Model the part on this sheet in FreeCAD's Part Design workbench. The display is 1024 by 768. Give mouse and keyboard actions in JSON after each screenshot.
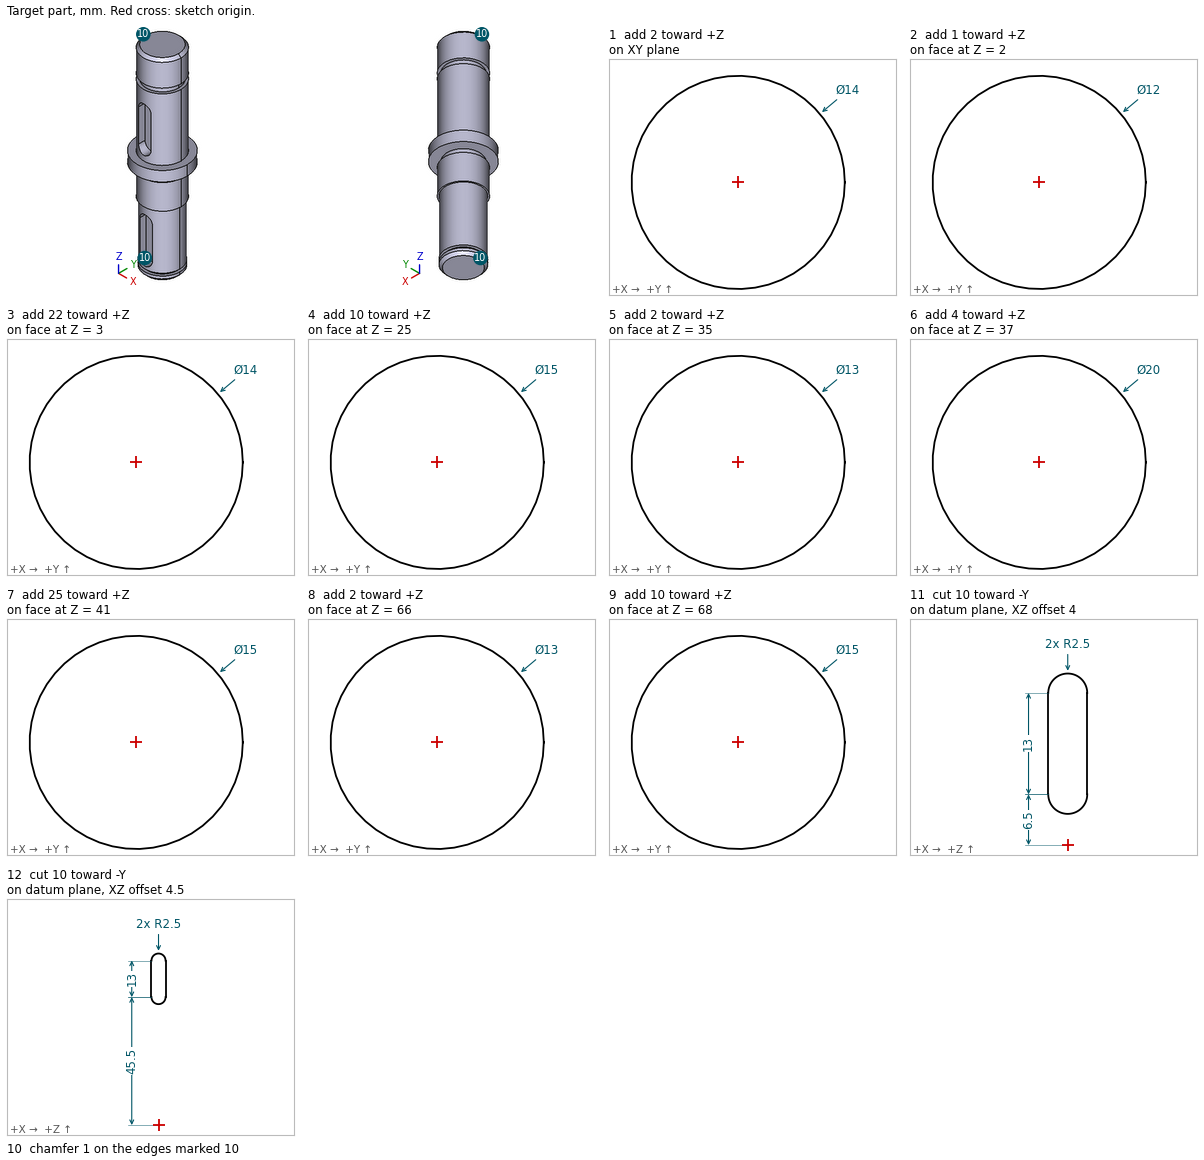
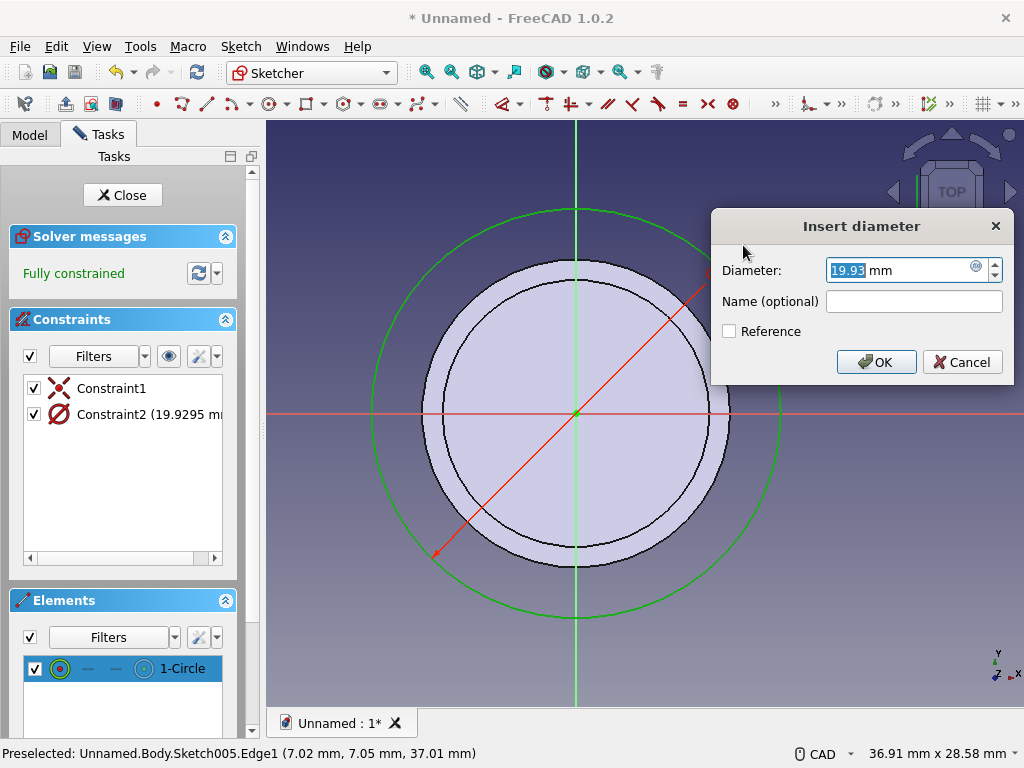
{"action": "type", "text": "20"}
{"action": "key", "text": "Return"}
{"action": "key", "text": "Escape"}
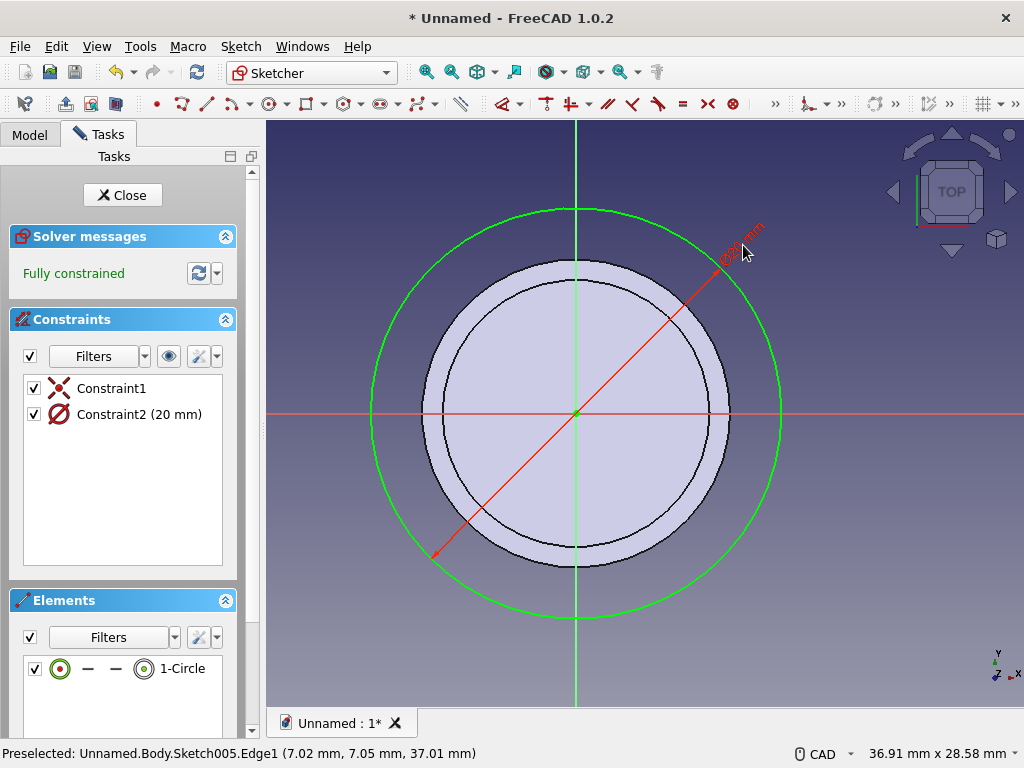
{"action": "left_click", "coordinate": [123, 195]}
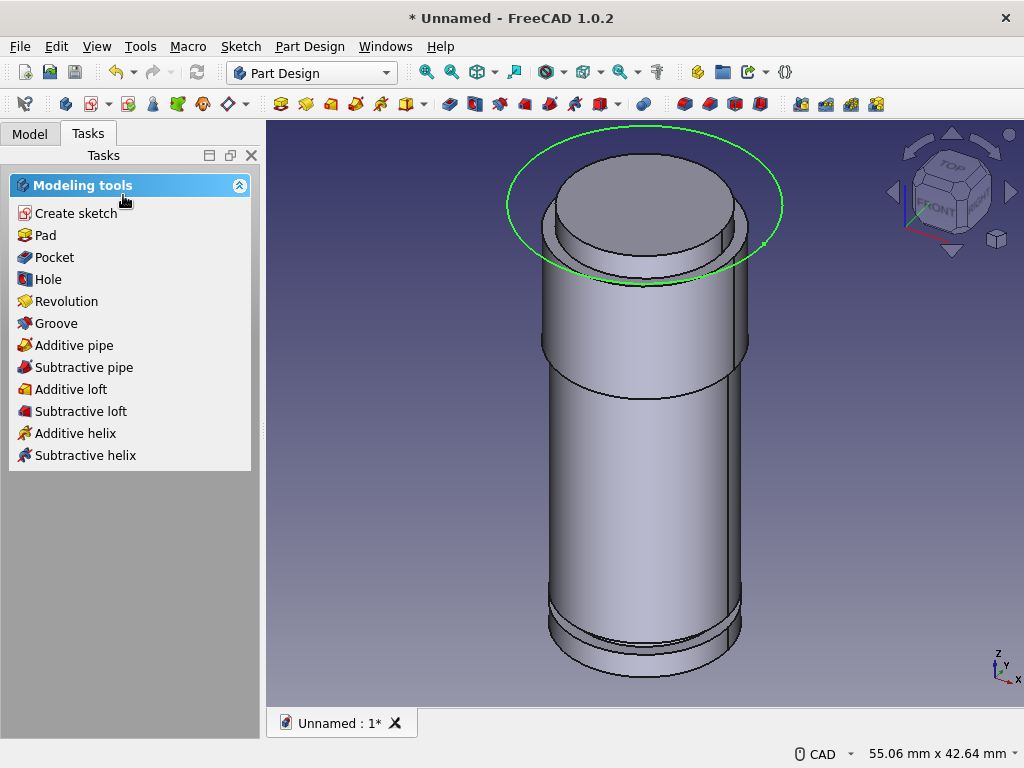
{"action": "left_click", "coordinate": [281, 104]}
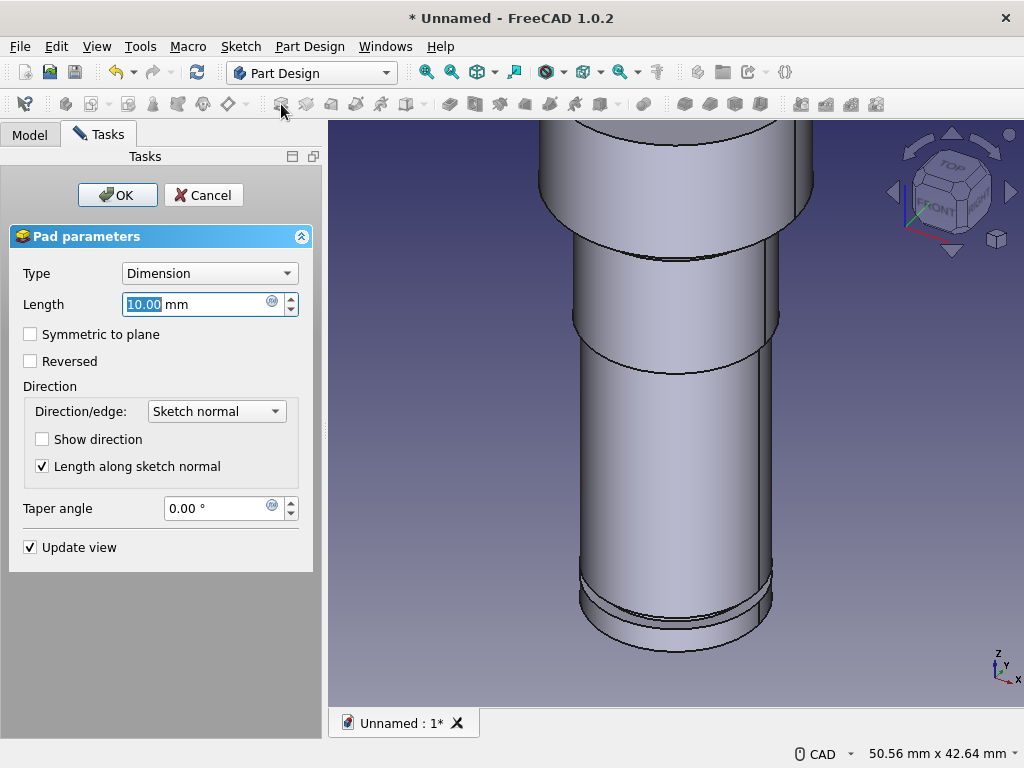
{"action": "type", "text": "4"}
{"action": "key", "text": "Tab"}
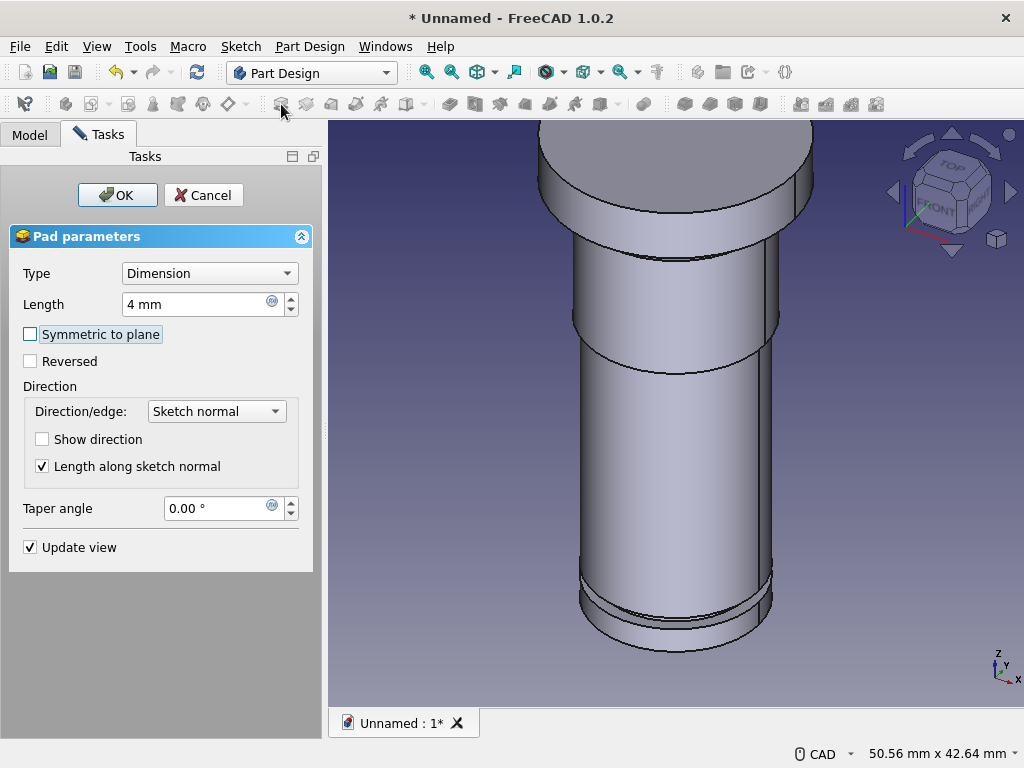
{"action": "left_click", "coordinate": [118, 195]}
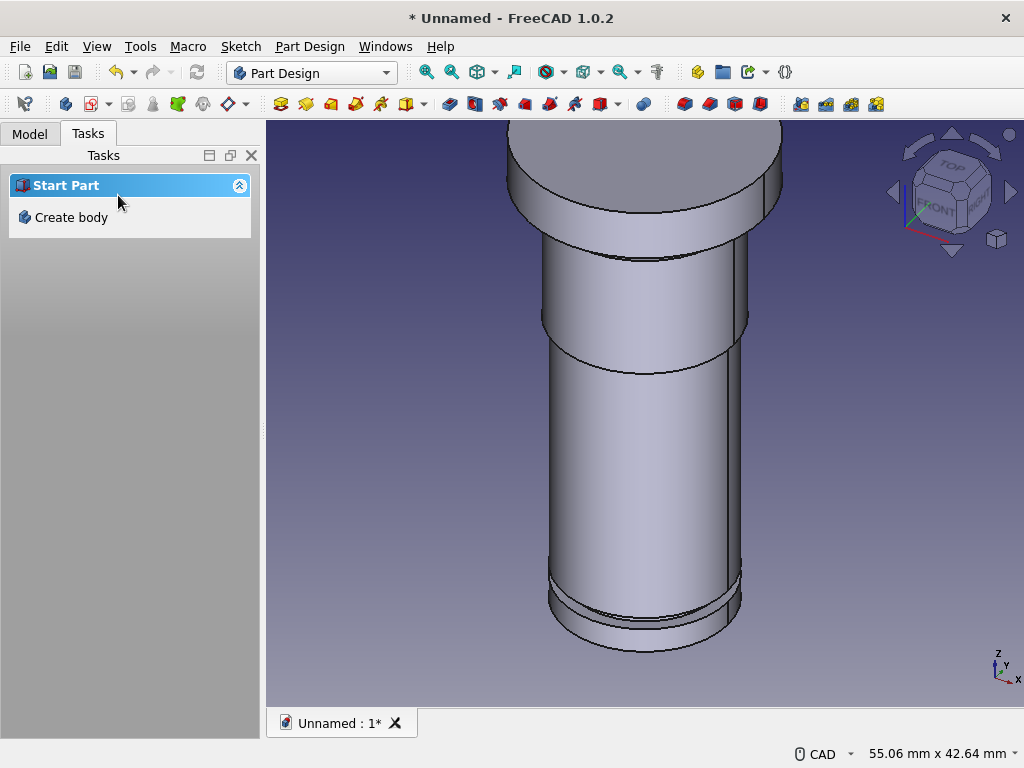
{"action": "left_click", "coordinate": [427, 72]}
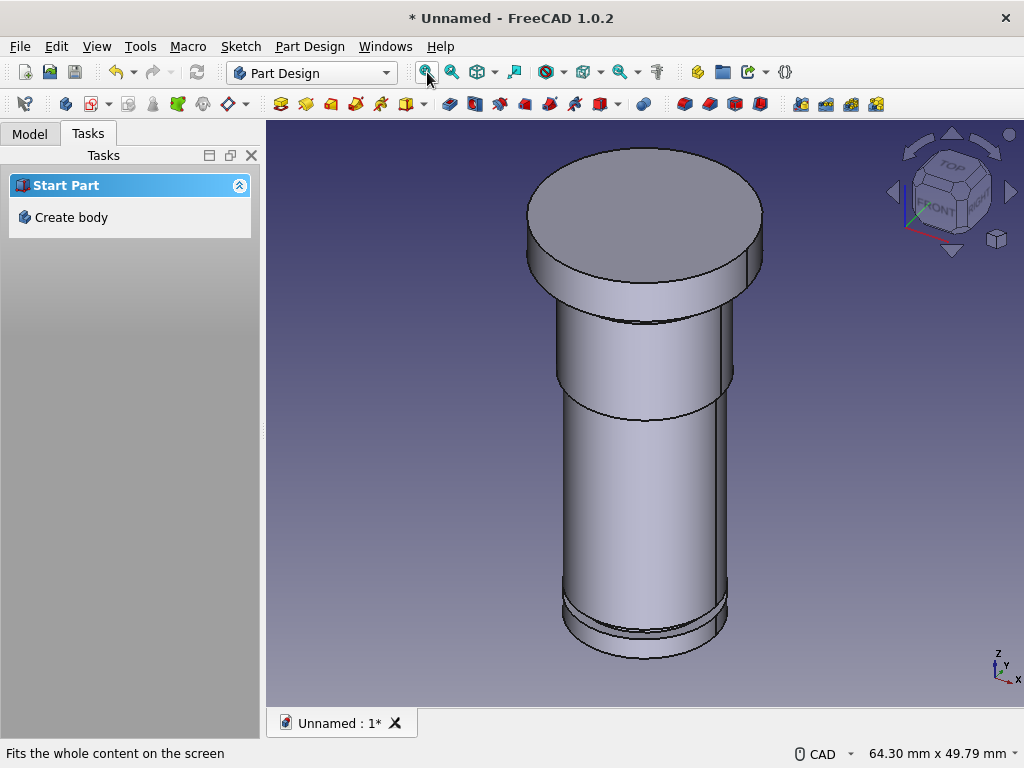
{"action": "left_click", "coordinate": [645, 214]}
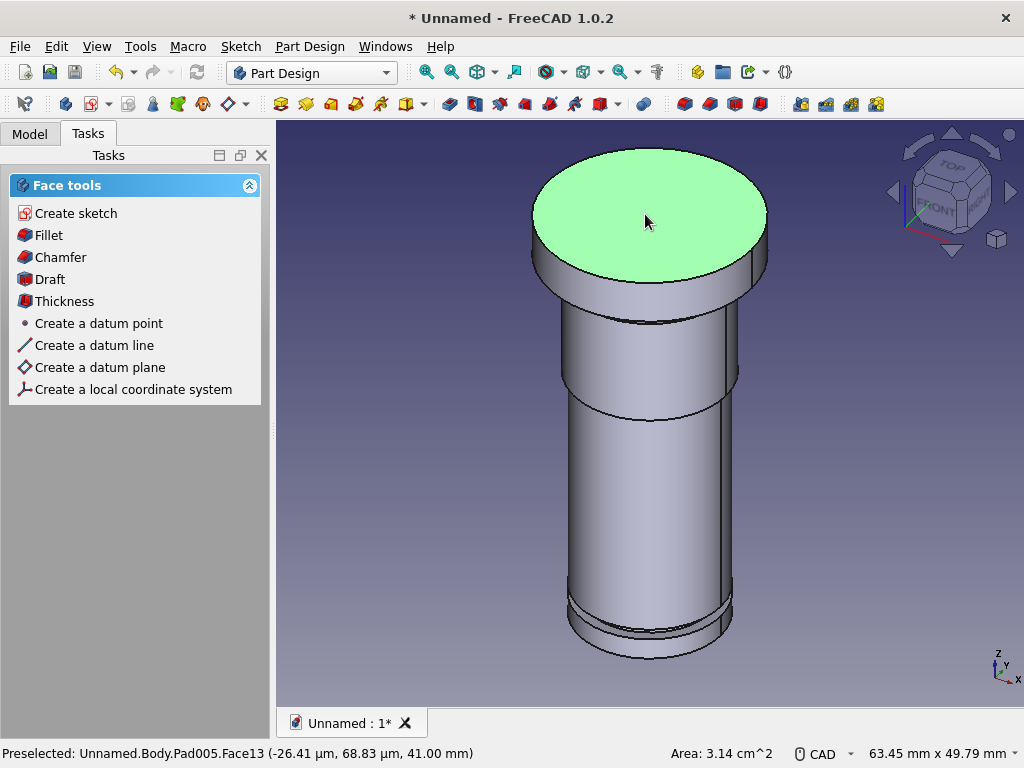
{"action": "left_click", "coordinate": [90, 104]}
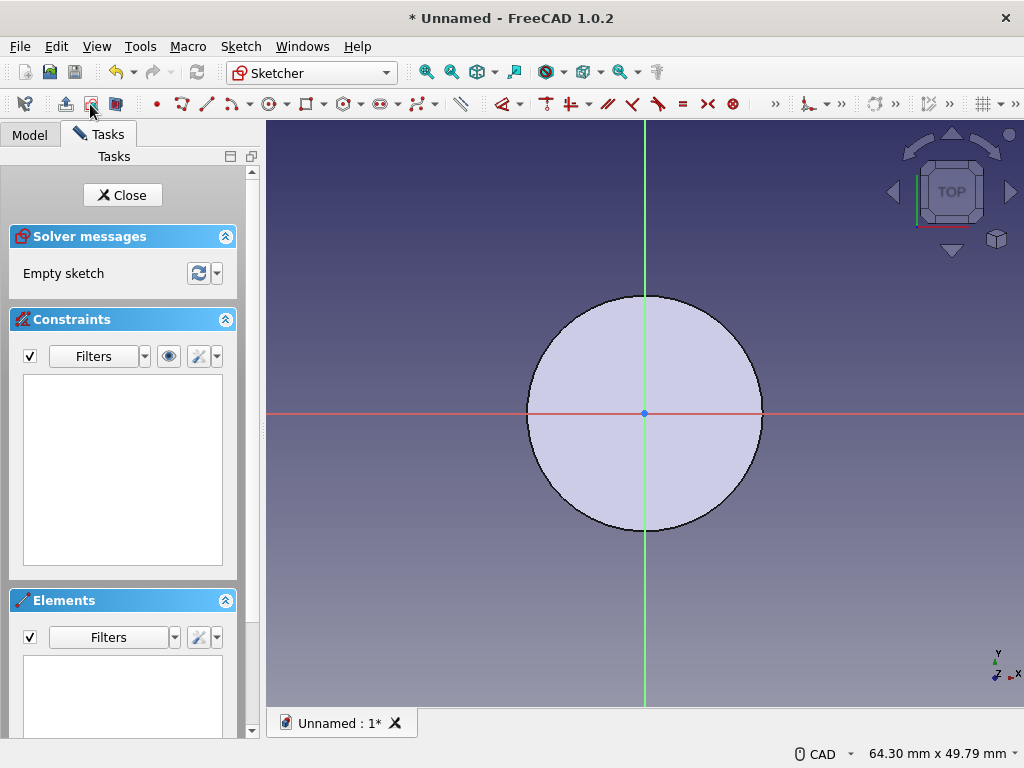
{"action": "scroll", "coordinate": [701, 413], "scroll_direction": "up", "scroll_amount": 4}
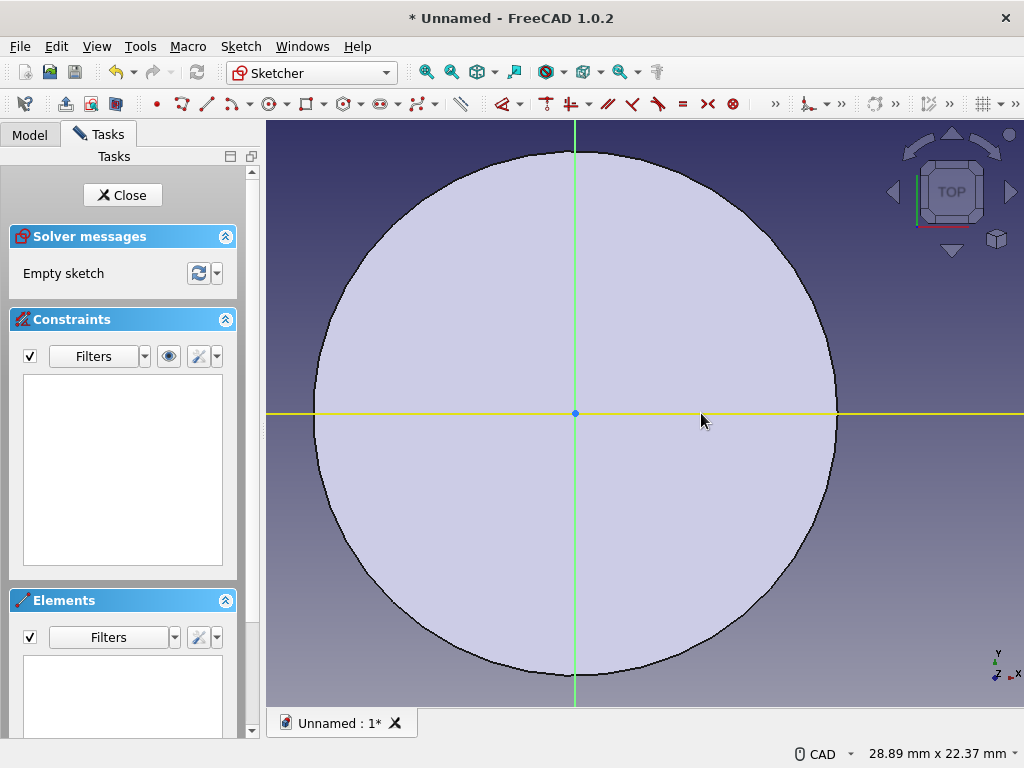
{"action": "left_click", "coordinate": [268, 104]}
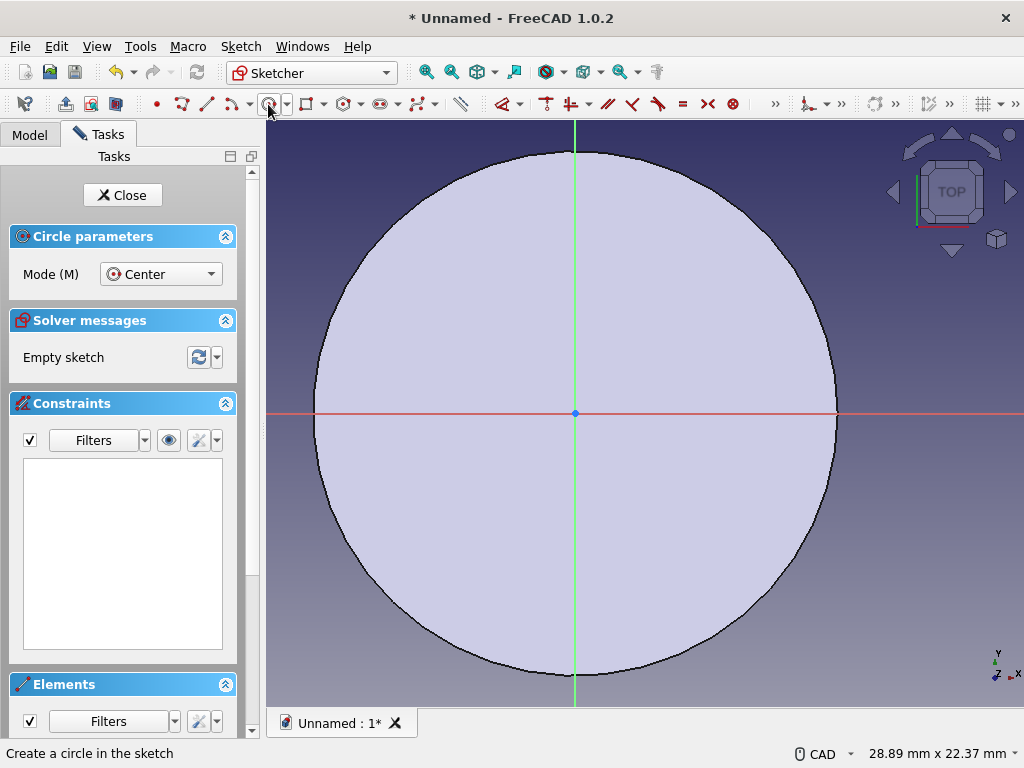
{"action": "left_click", "coordinate": [575, 414]}
{"action": "left_click", "coordinate": [714, 274]}
{"action": "key", "text": "Escape"}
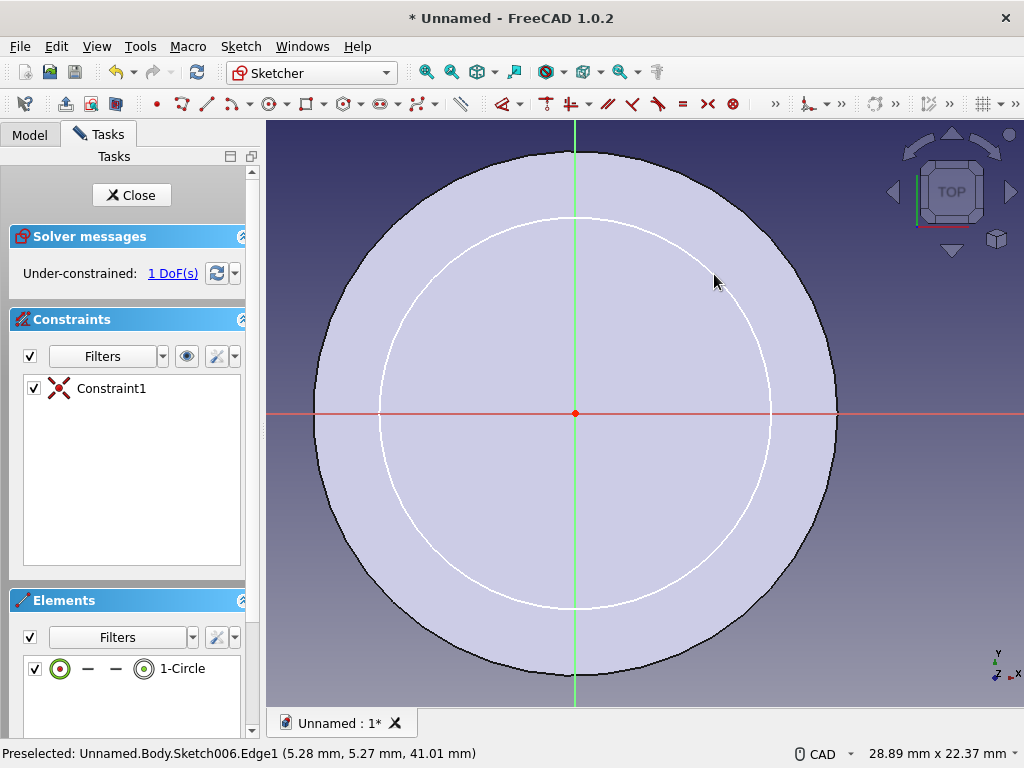
{"action": "left_click", "coordinate": [502, 104]}